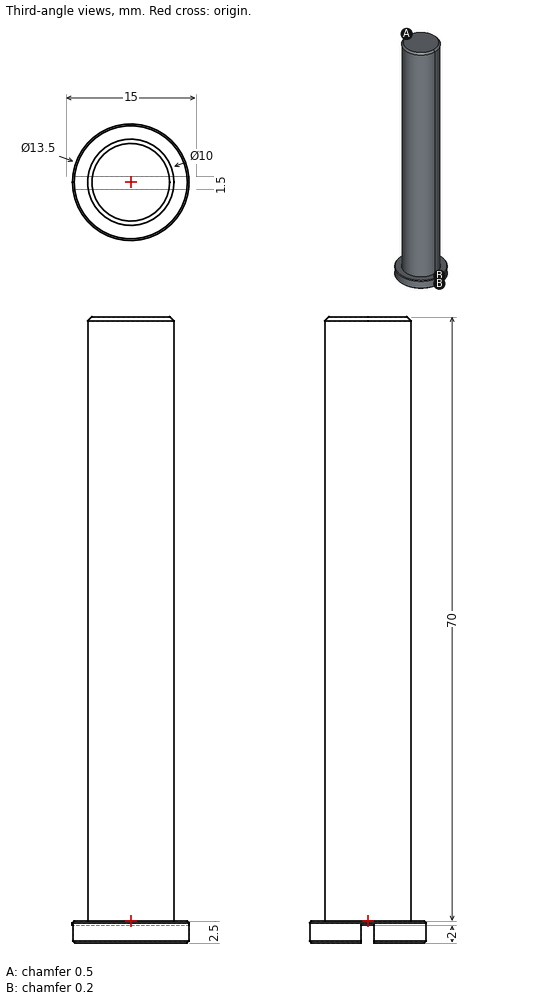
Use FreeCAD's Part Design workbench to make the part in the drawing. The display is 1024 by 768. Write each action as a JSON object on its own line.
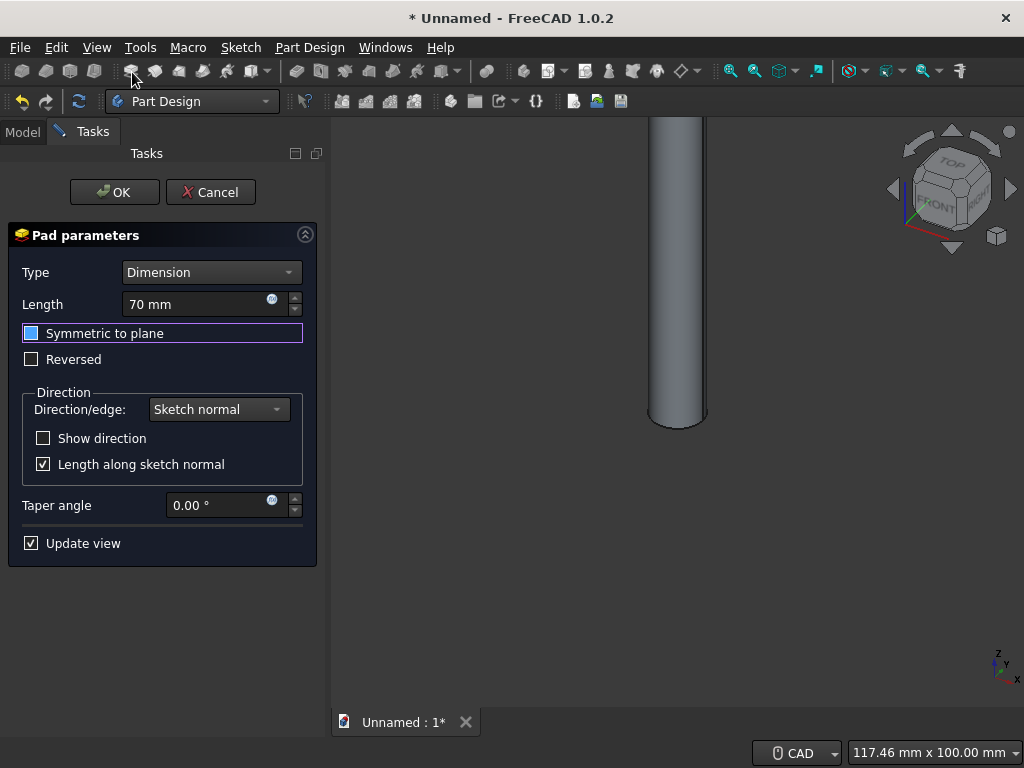
{"action": "left_click", "coordinate": [115, 192]}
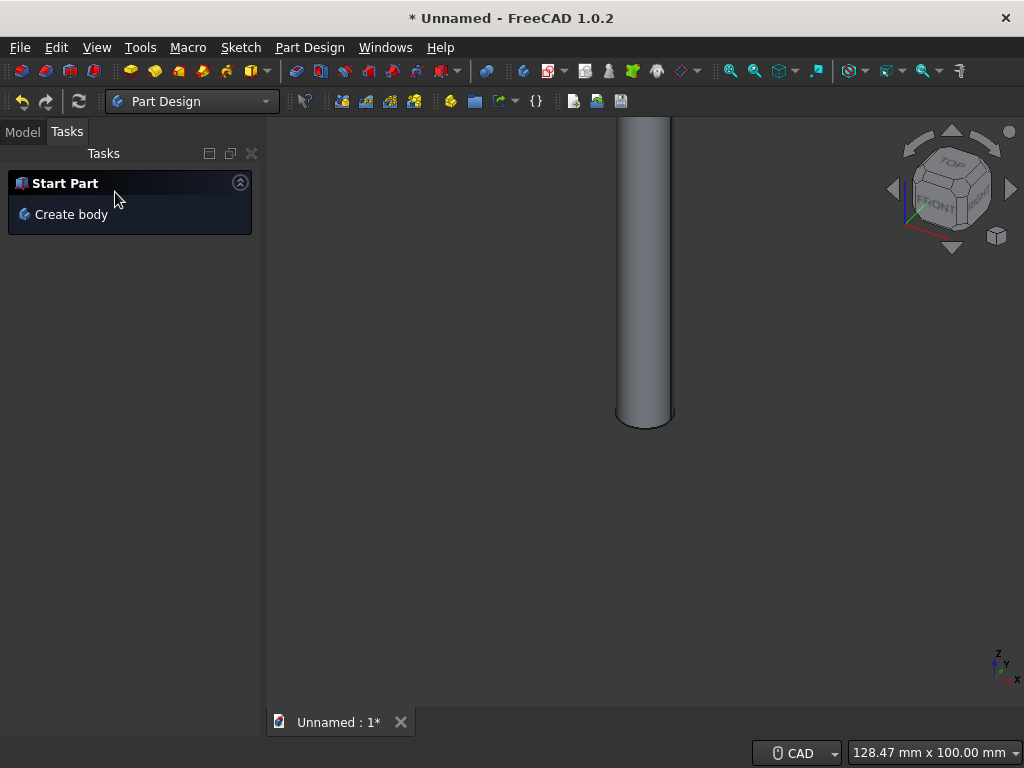
{"action": "left_click", "coordinate": [732, 72]}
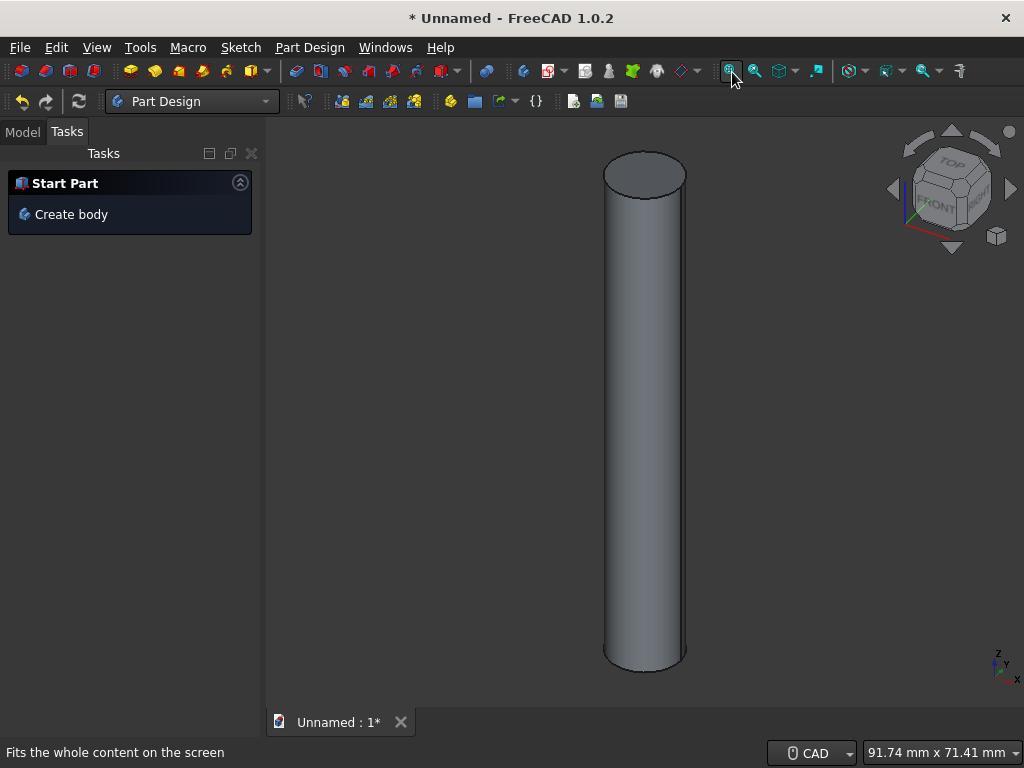
{"action": "left_click", "coordinate": [548, 72]}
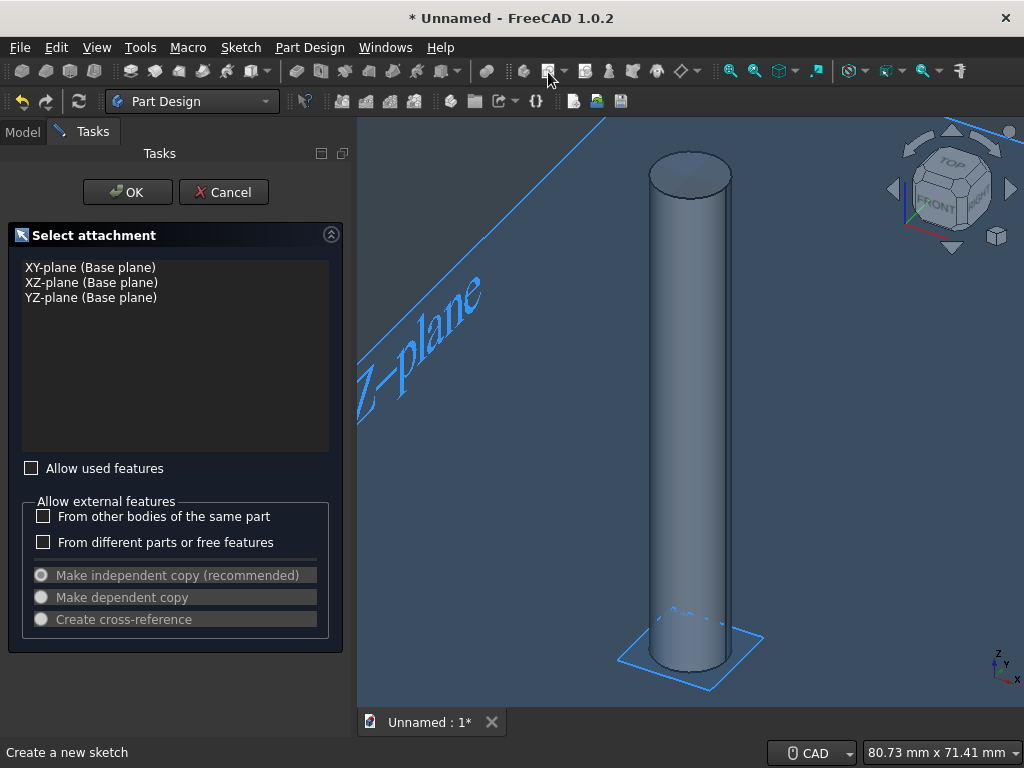
{"action": "left_click", "coordinate": [82, 268]}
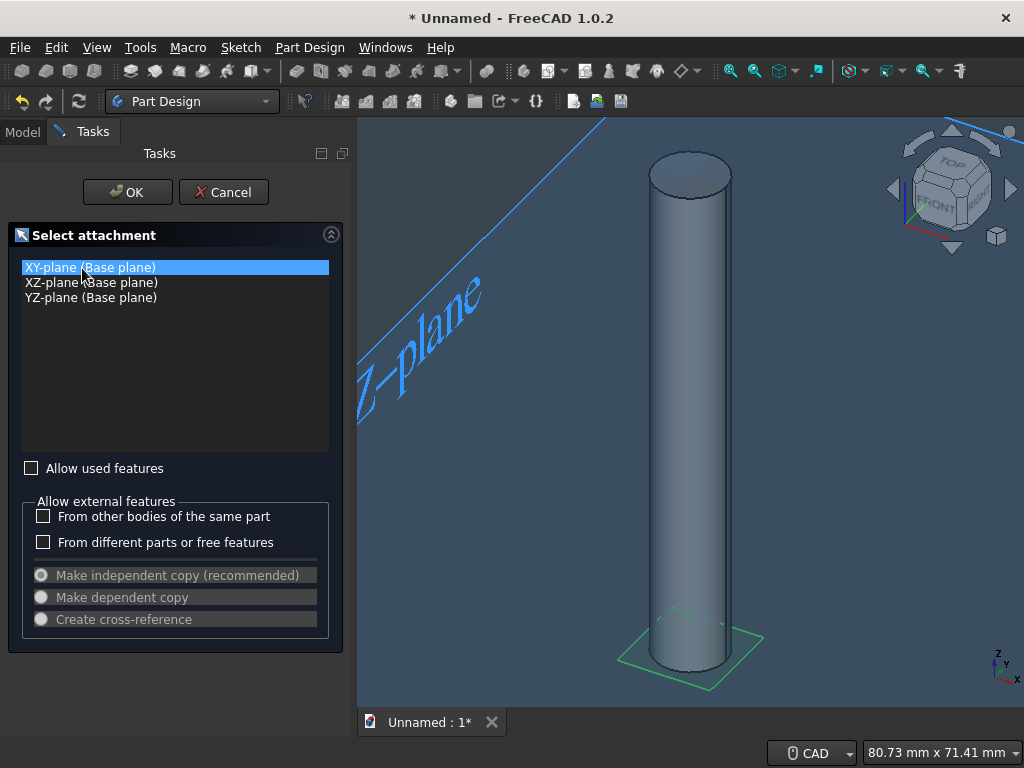
{"action": "left_click", "coordinate": [128, 192]}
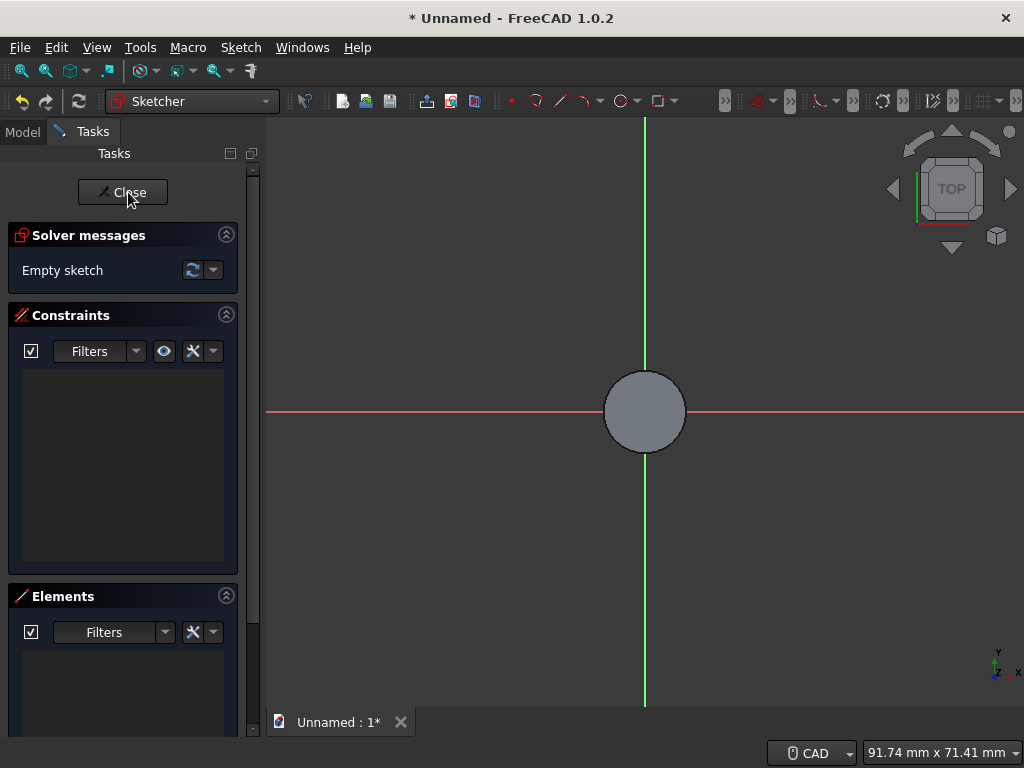
{"action": "left_click", "coordinate": [476, 102]}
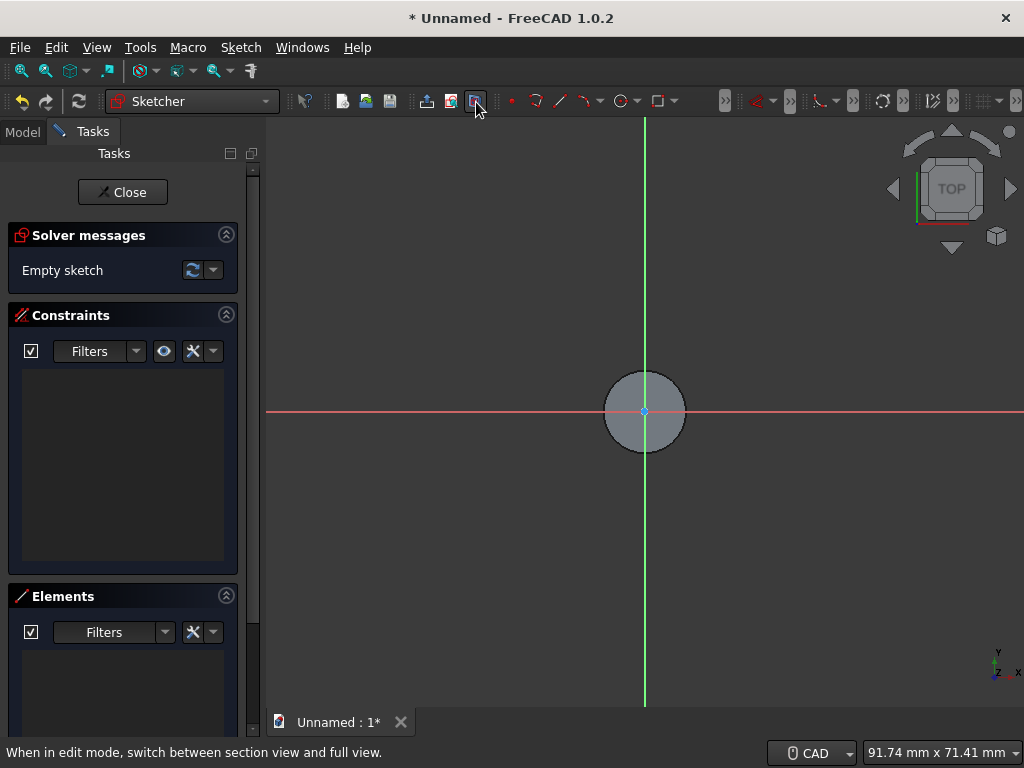
{"action": "scroll", "coordinate": [674, 412], "scroll_direction": "up", "scroll_amount": 6}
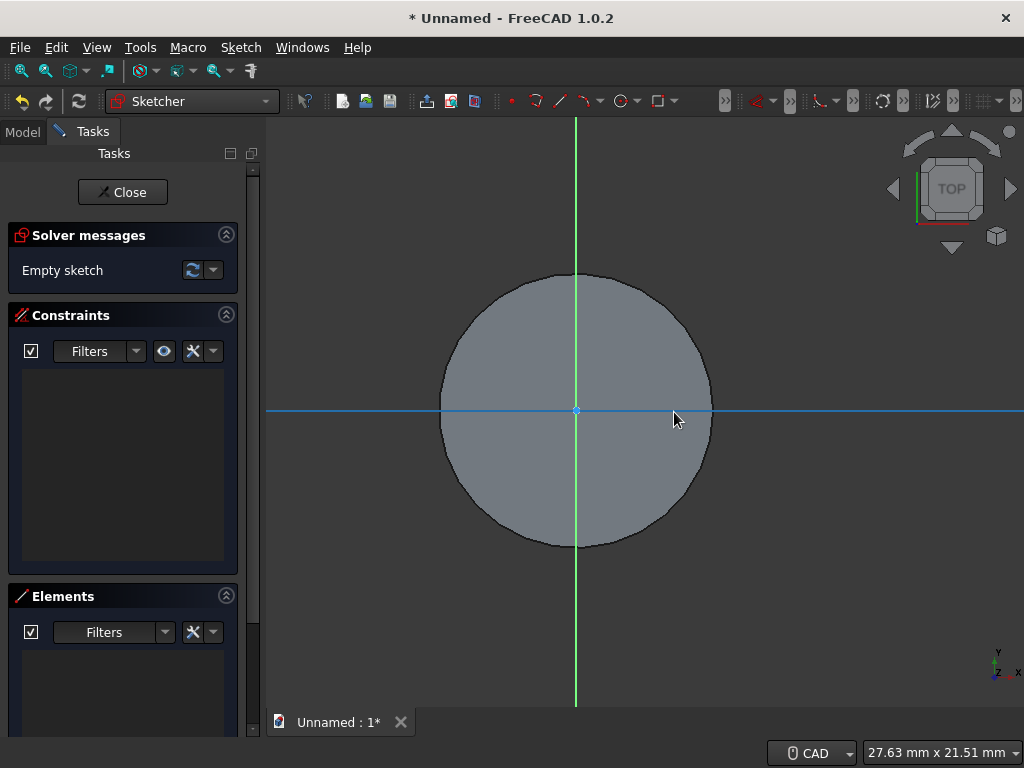
{"action": "left_click", "coordinate": [622, 102]}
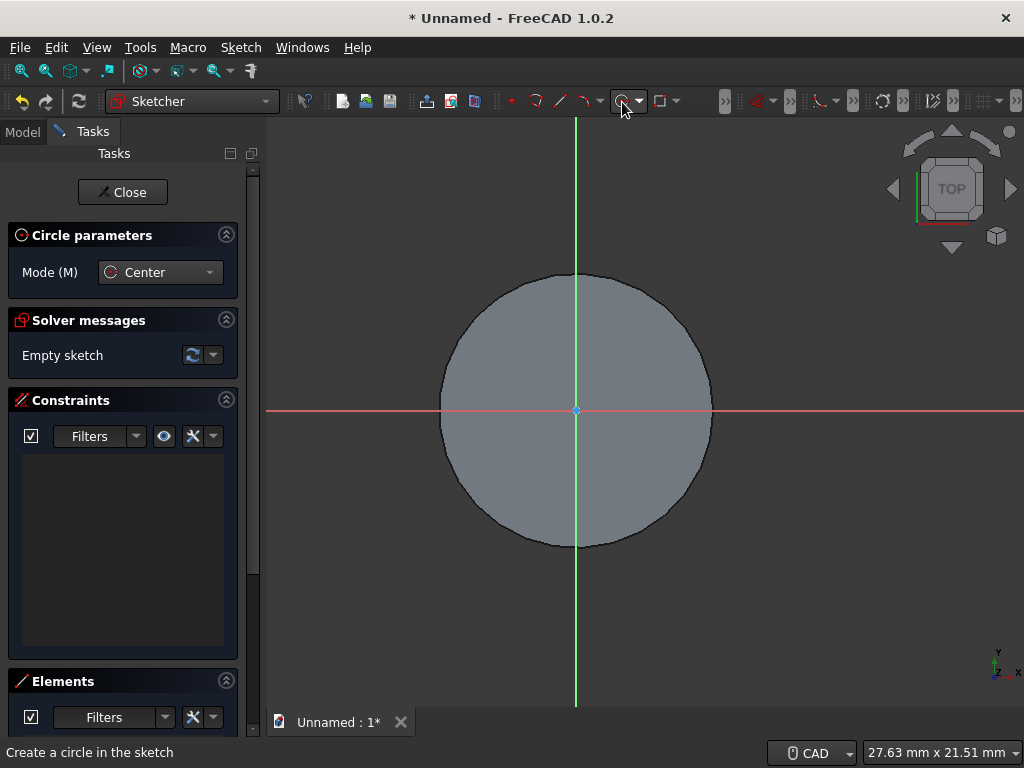
{"action": "left_click", "coordinate": [576, 411]}
{"action": "left_click", "coordinate": [707, 280]}
{"action": "key", "text": "Escape"}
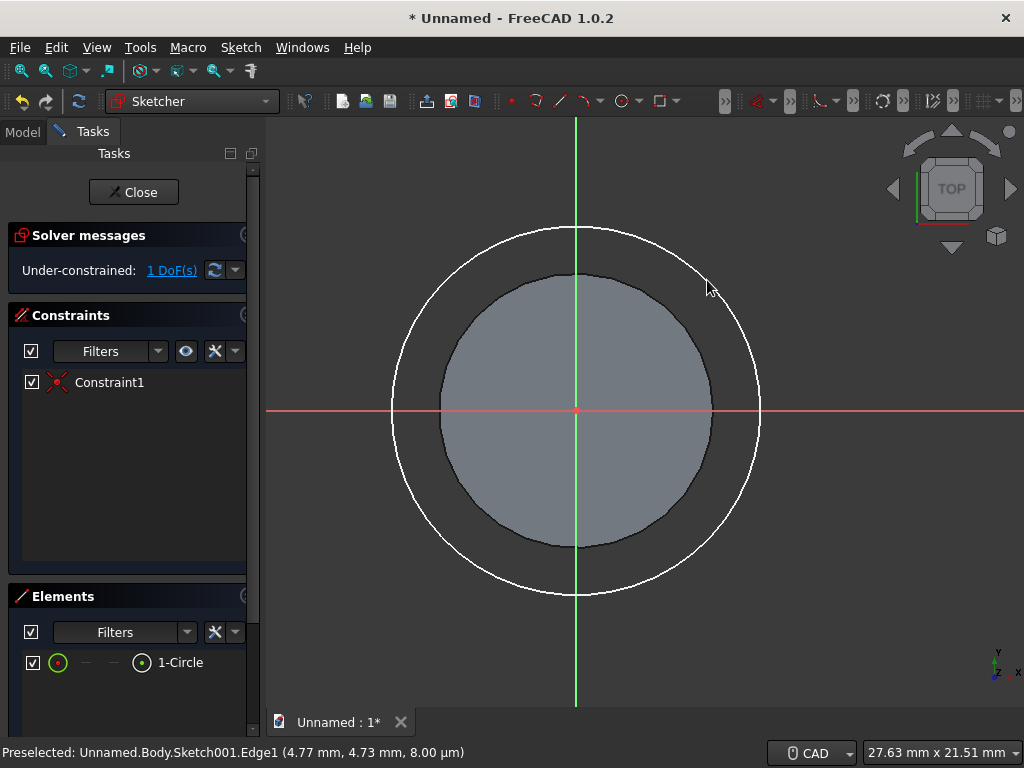
{"action": "left_click", "coordinate": [756, 102]}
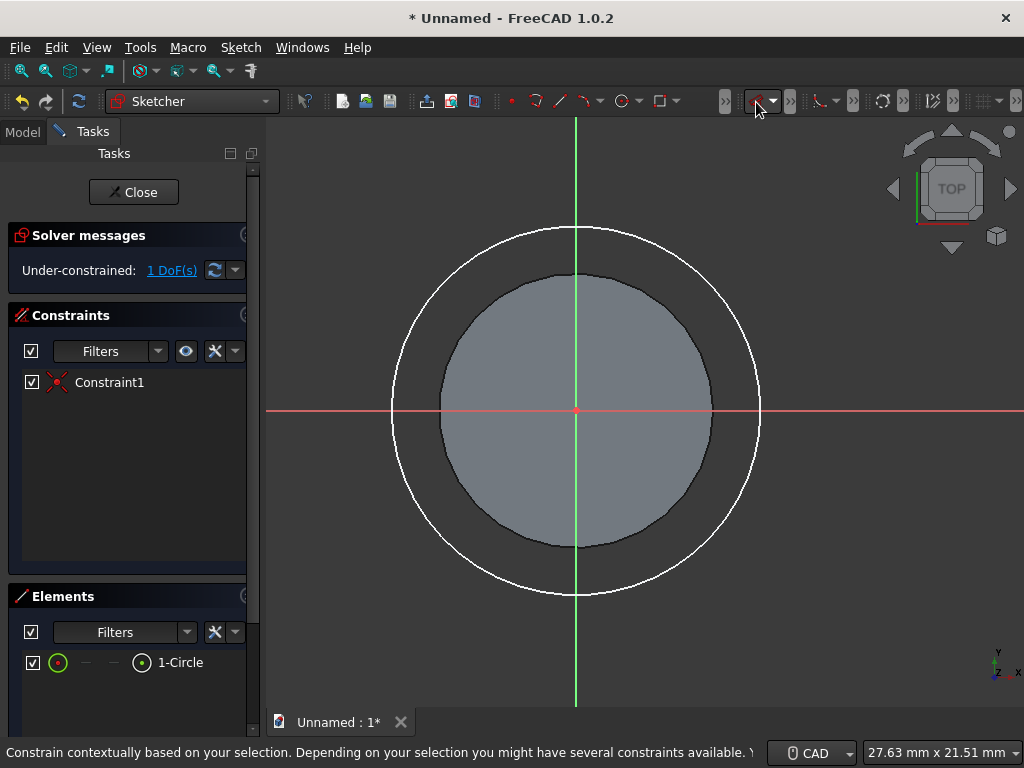
{"action": "left_click", "coordinate": [706, 280]}
{"action": "left_click", "coordinate": [729, 257]}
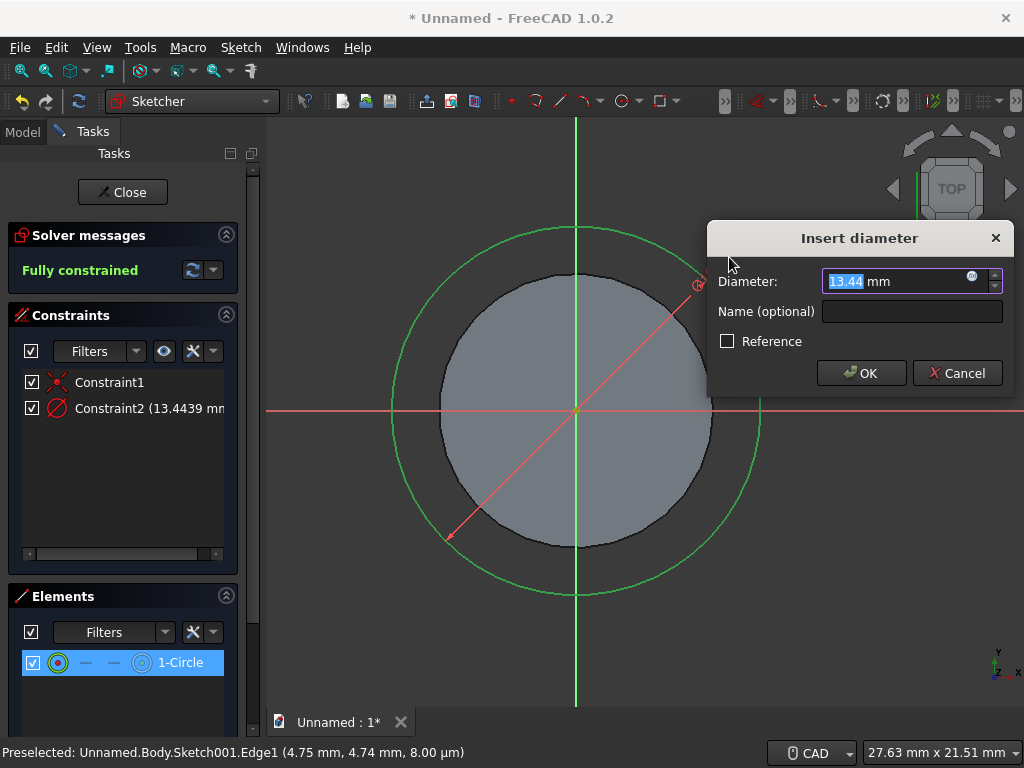
{"action": "type", "text": "13.5"}
{"action": "key", "text": "Return"}
{"action": "key", "text": "Escape"}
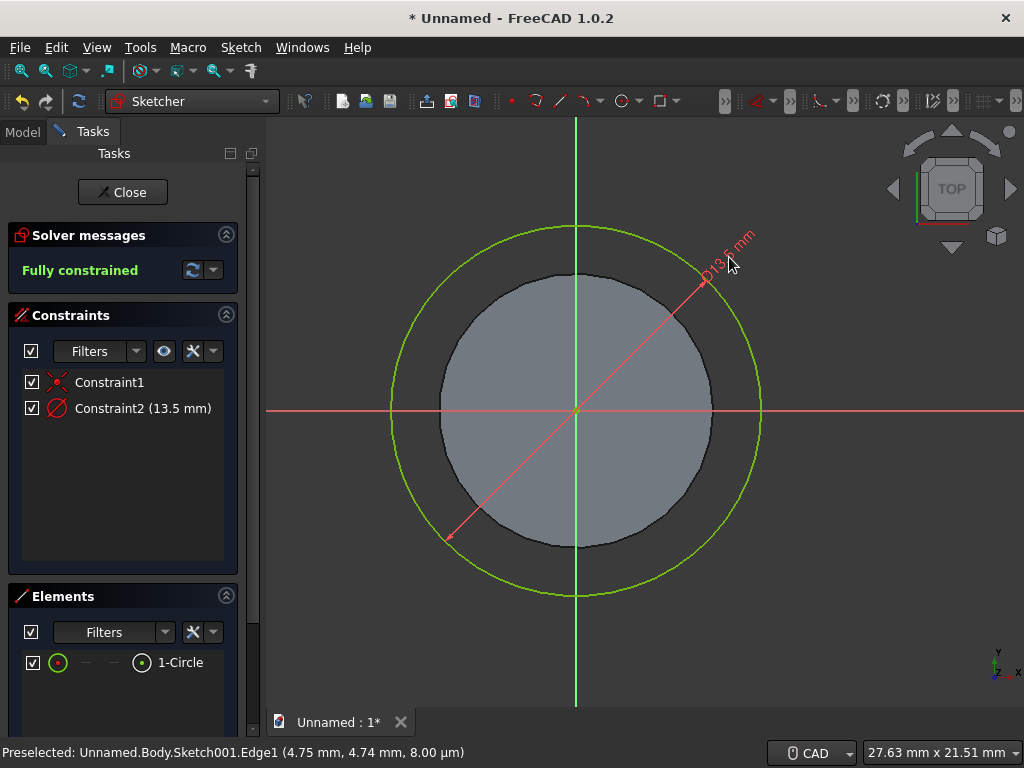
{"action": "left_click", "coordinate": [123, 192]}